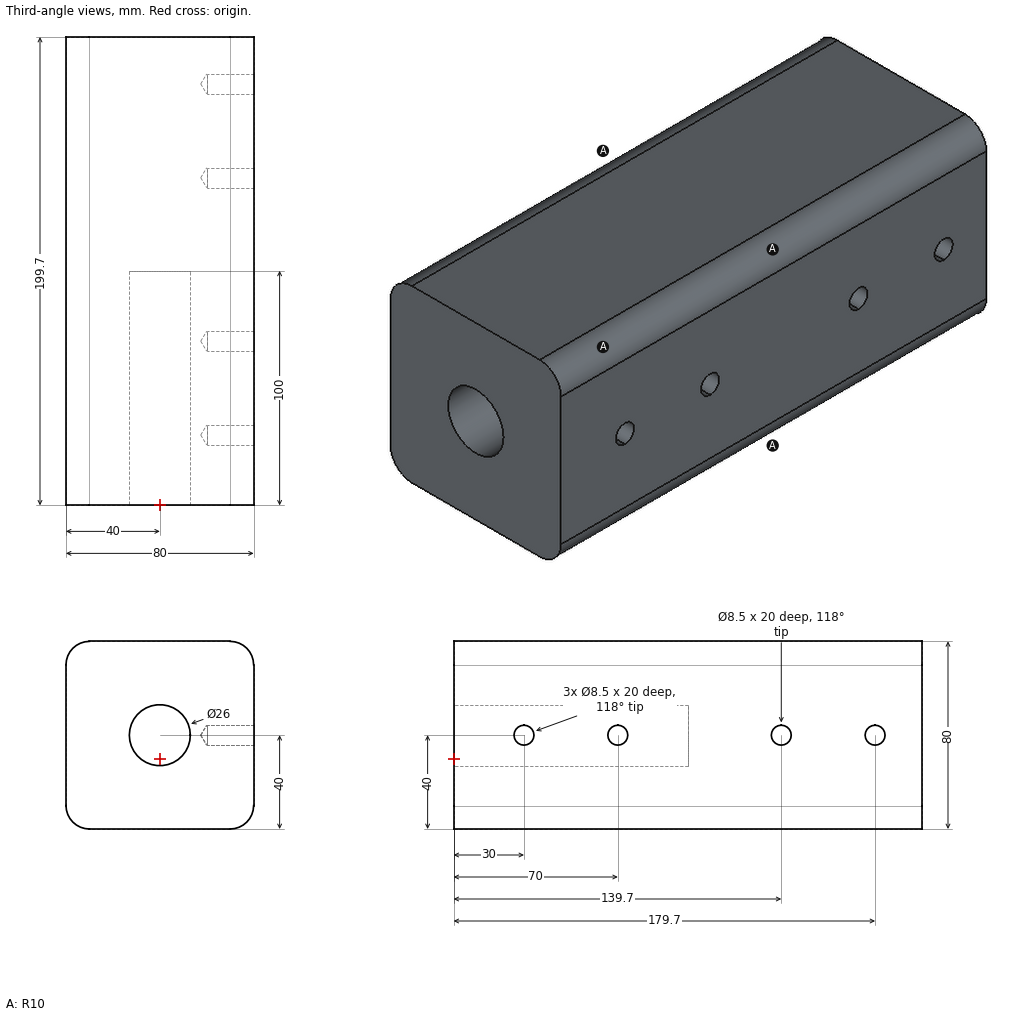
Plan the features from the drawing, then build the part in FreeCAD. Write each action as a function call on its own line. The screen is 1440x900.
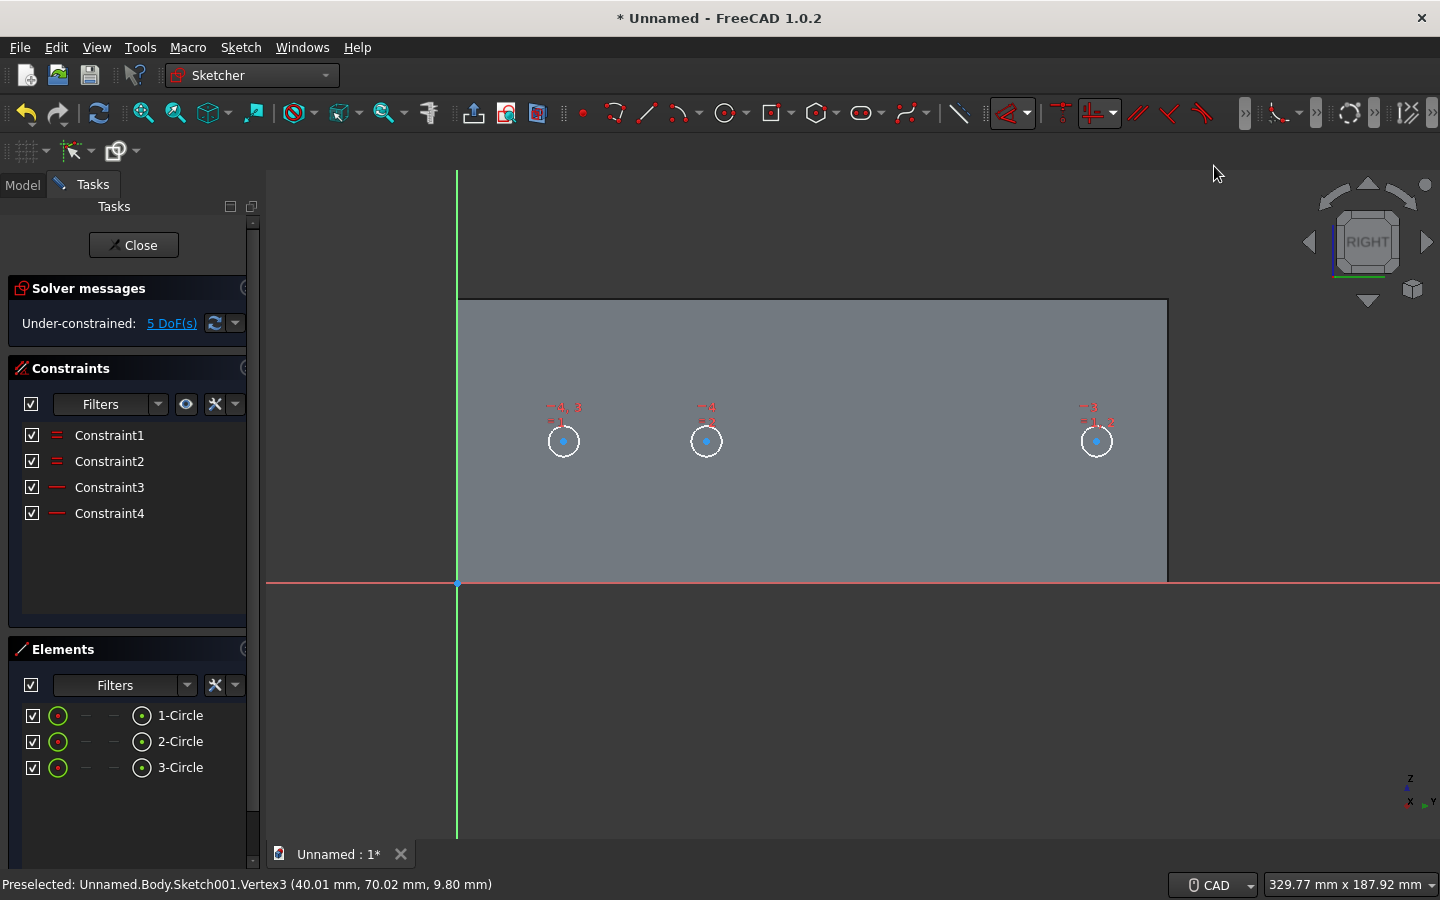
scroll(574, 431, up, 2)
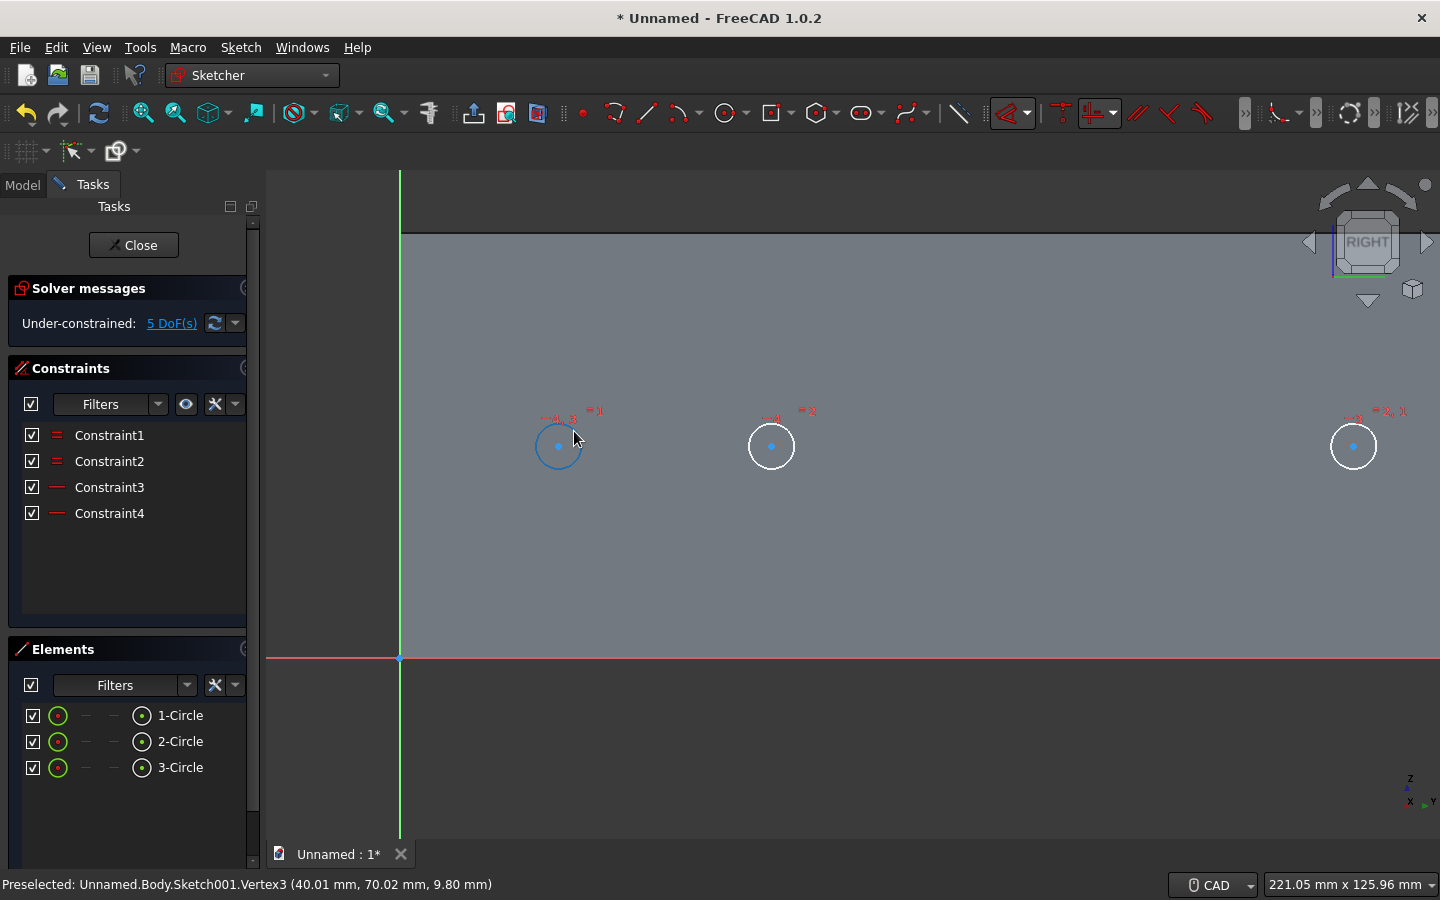
click(575, 430)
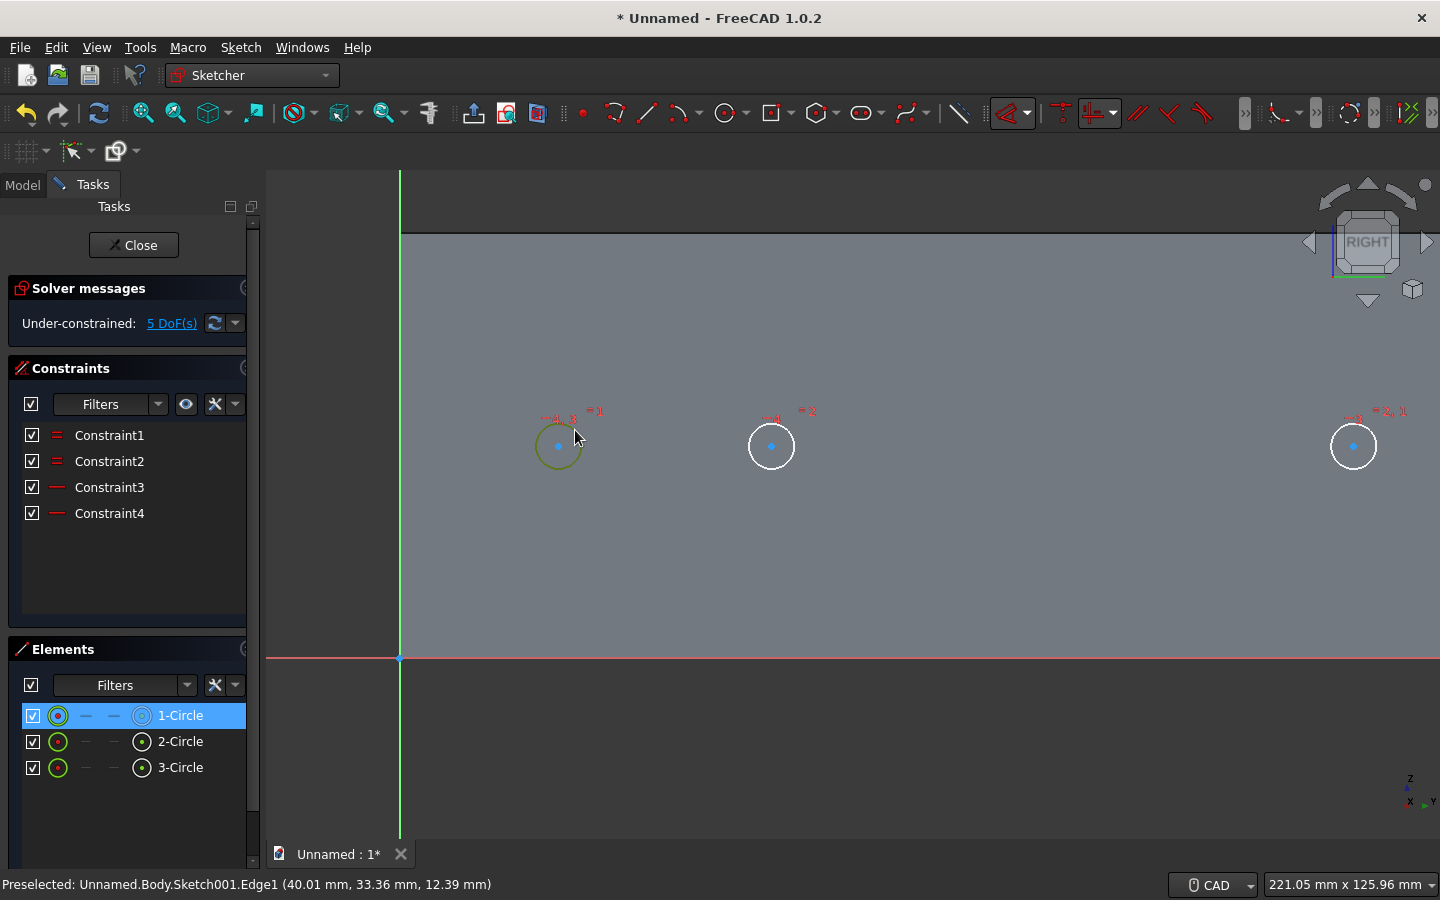
click(1030, 114)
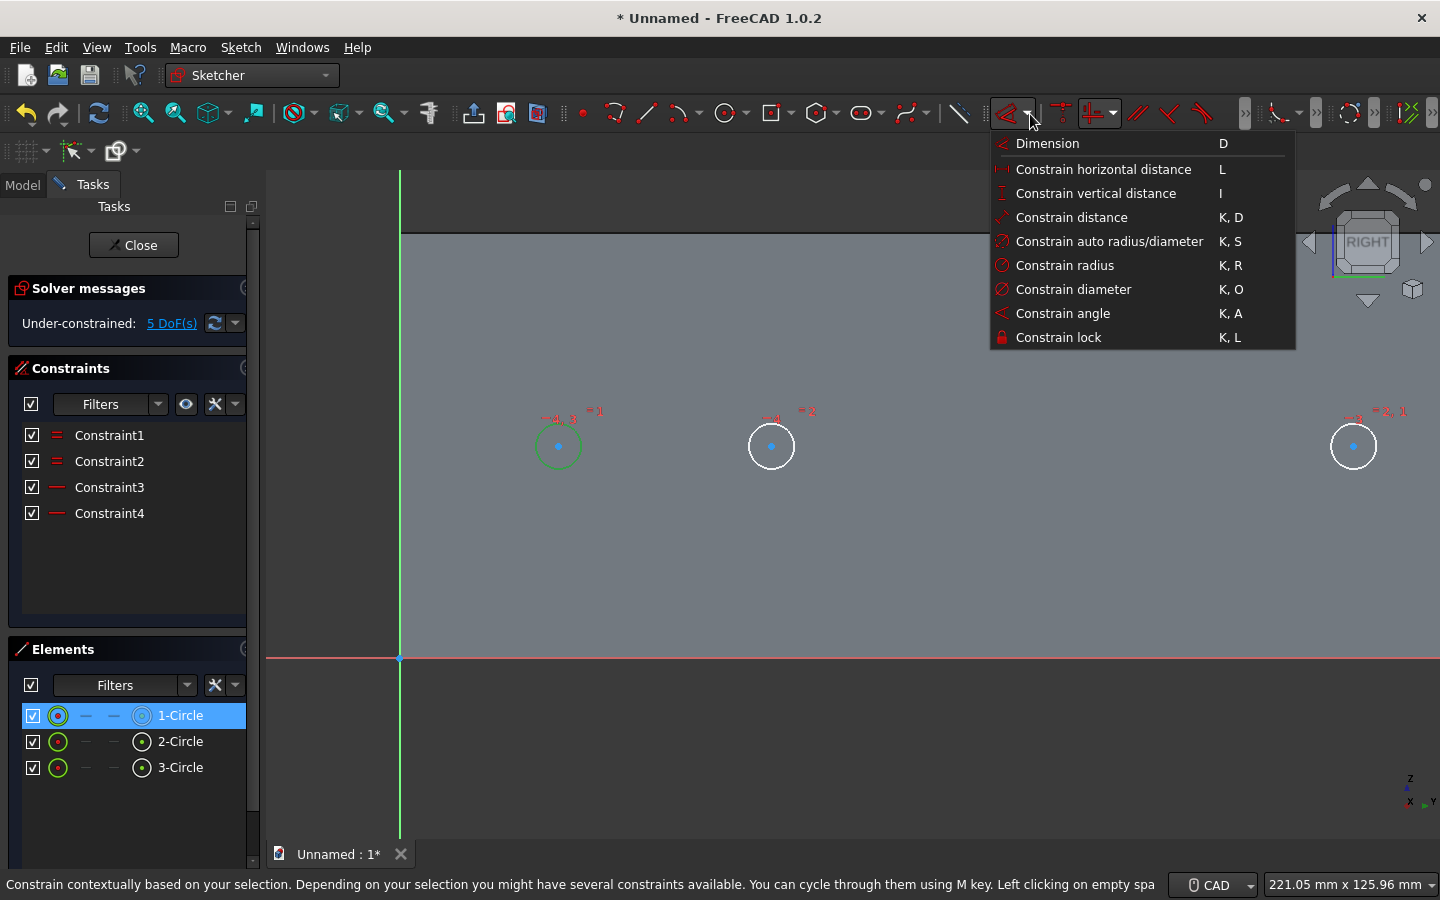
click(1143, 289)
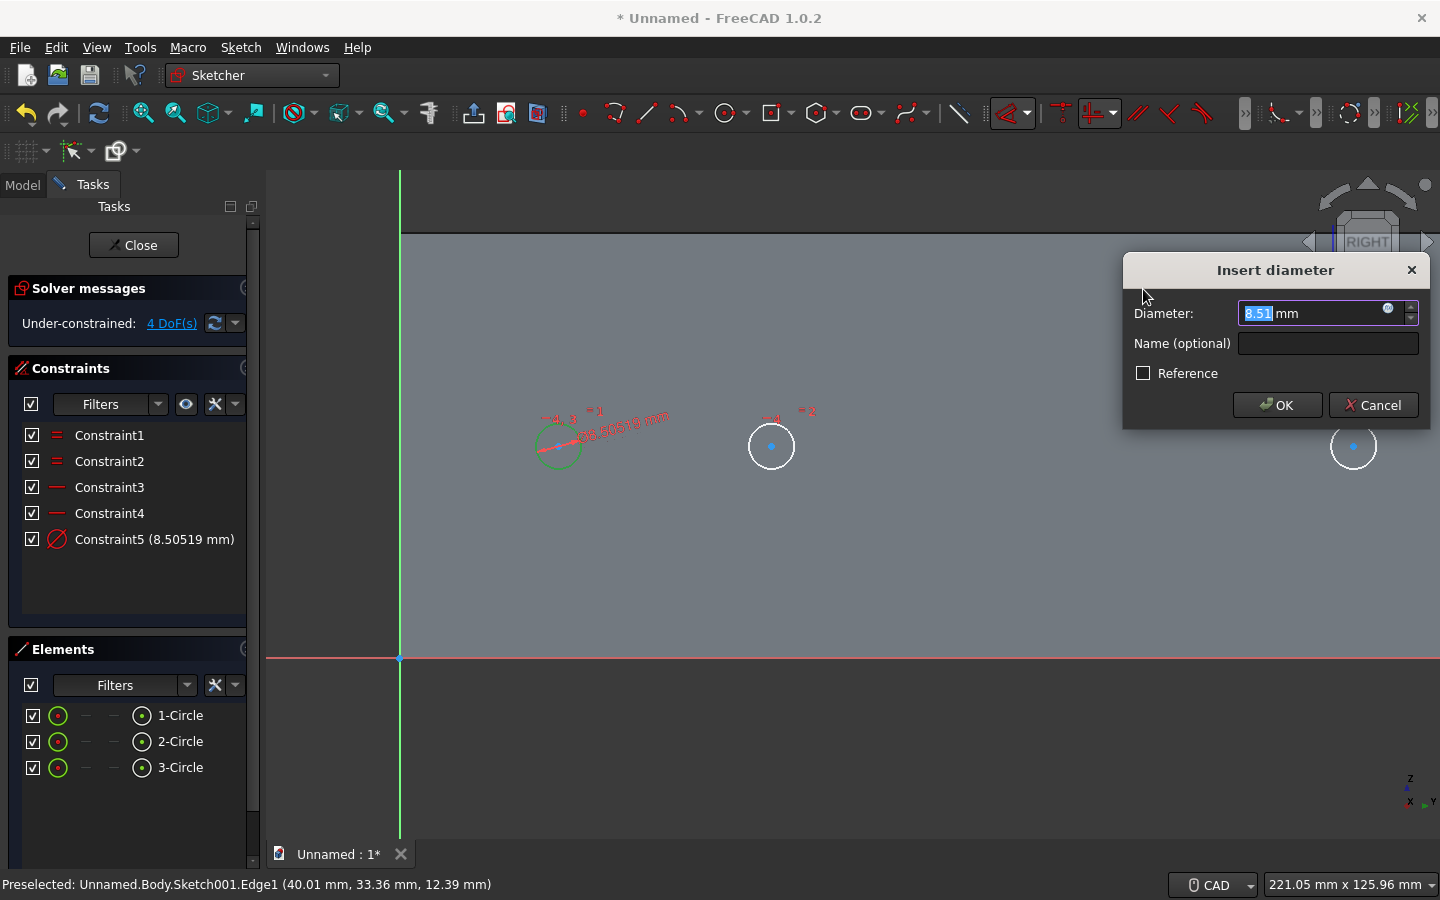
text(8.5)
key(Return)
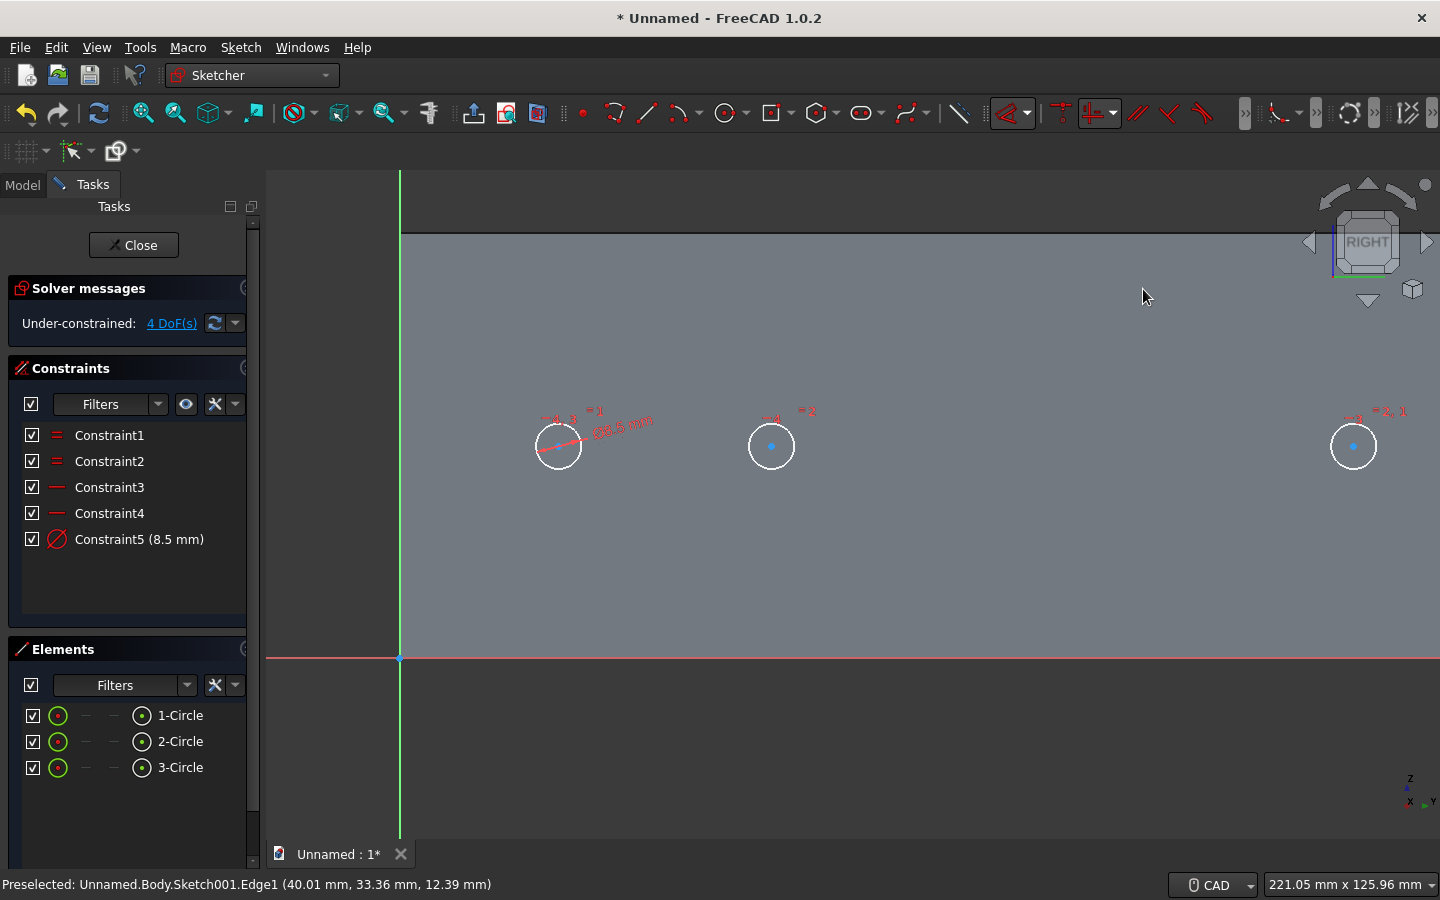
click(559, 446)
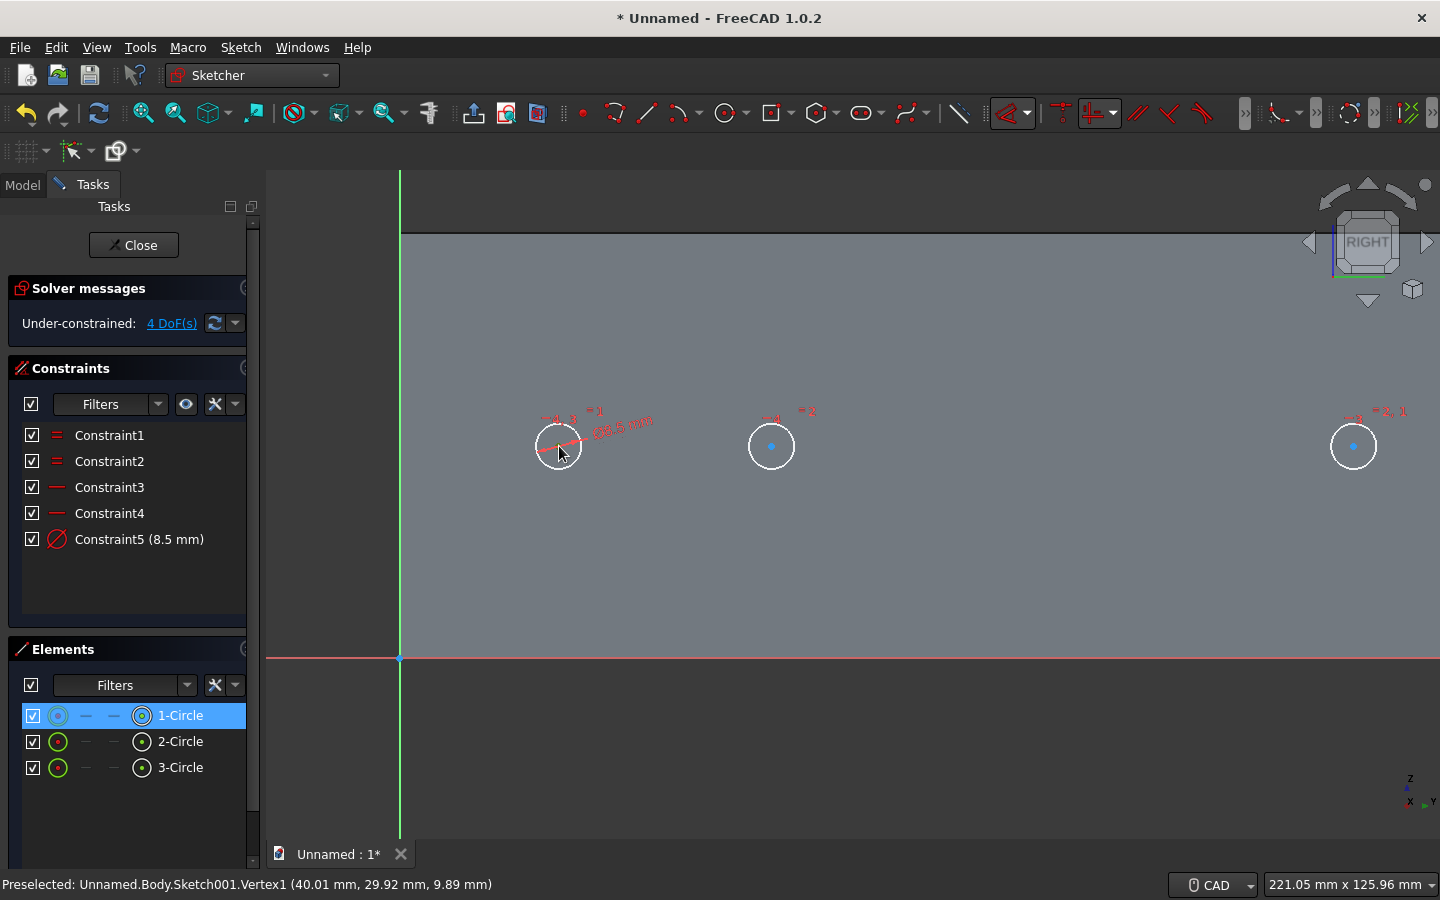
key(l)